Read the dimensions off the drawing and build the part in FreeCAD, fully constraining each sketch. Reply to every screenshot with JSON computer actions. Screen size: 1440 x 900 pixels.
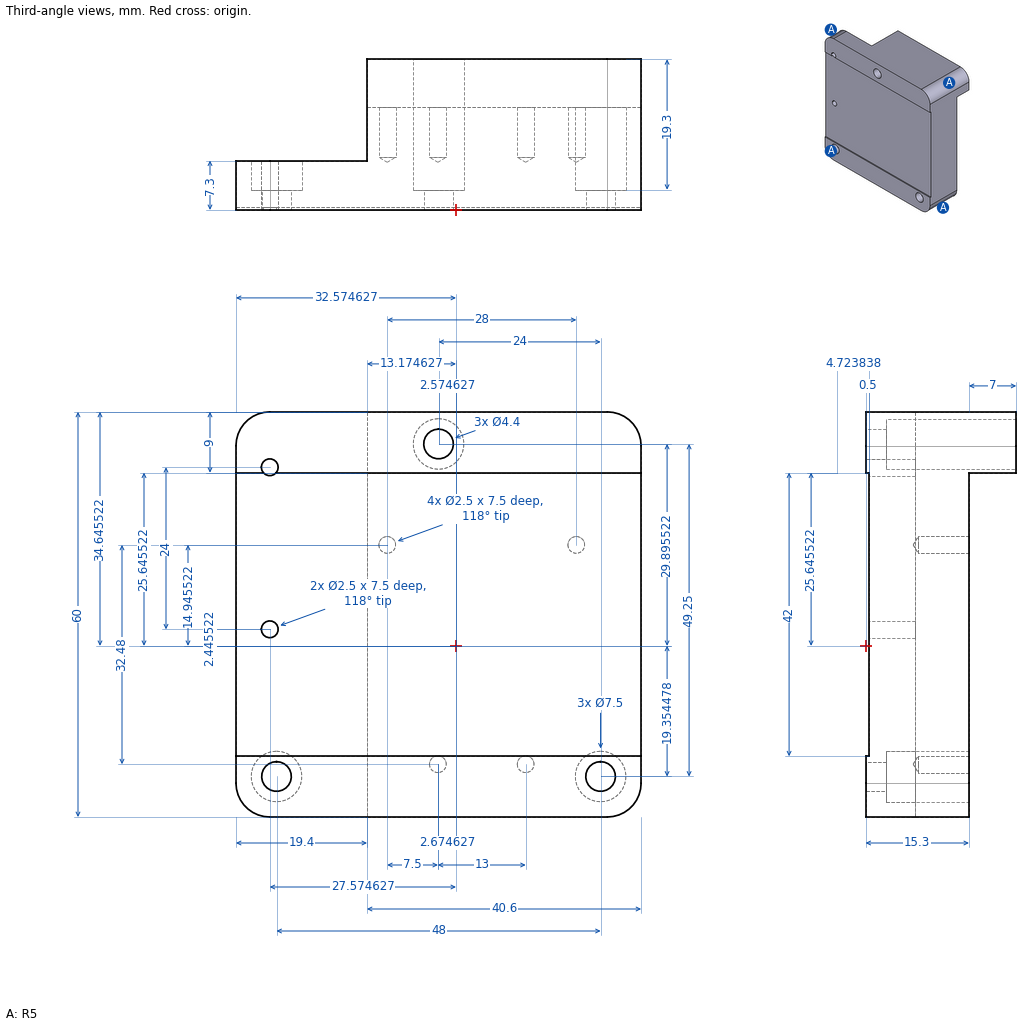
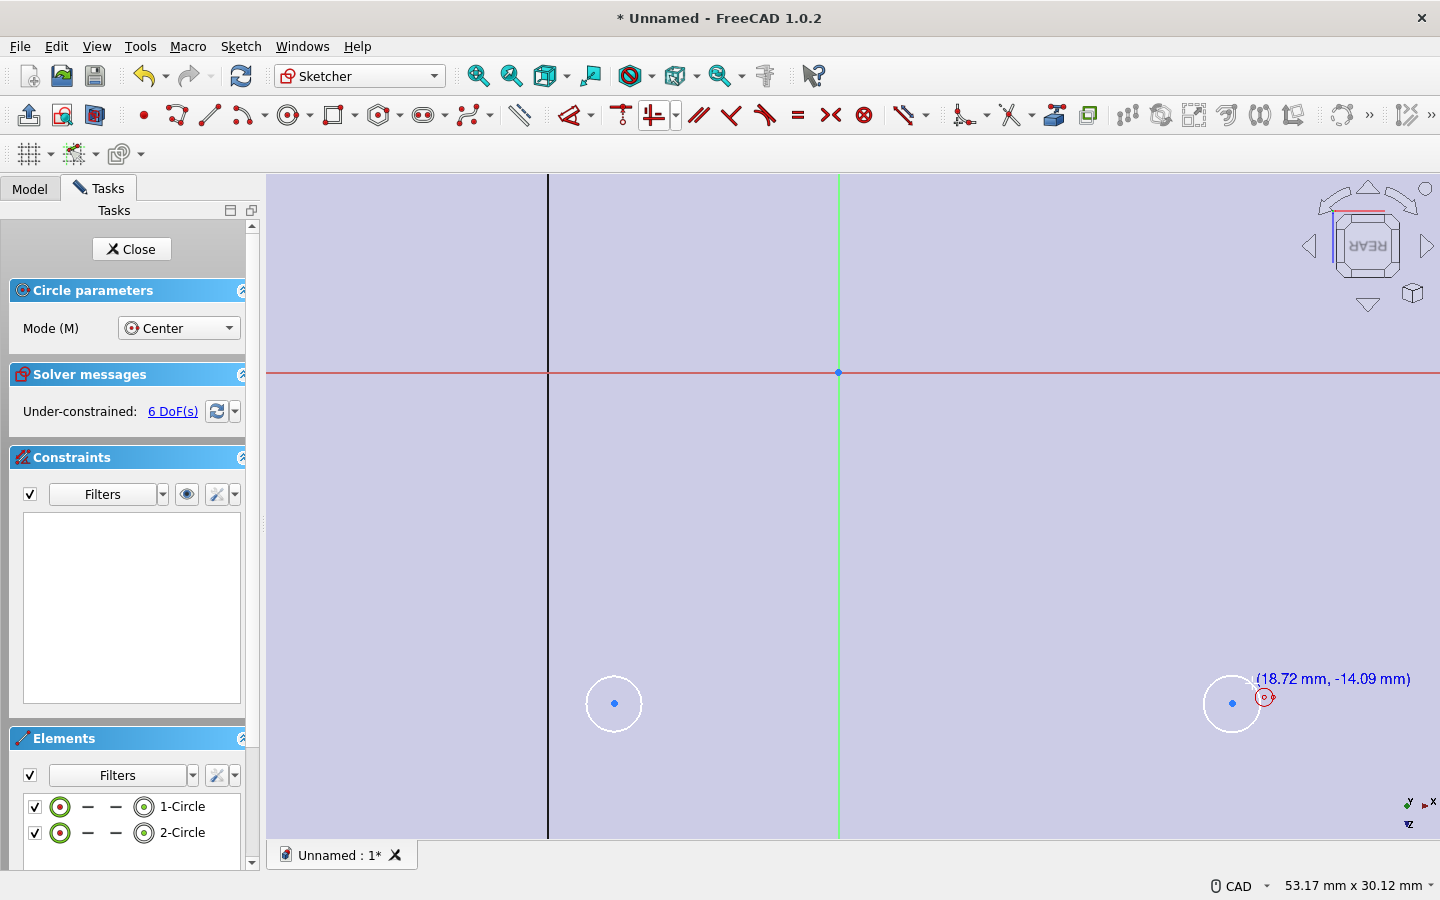
{"action": "scroll", "coordinate": [616, 704], "scroll_direction": "down", "scroll_amount": 3}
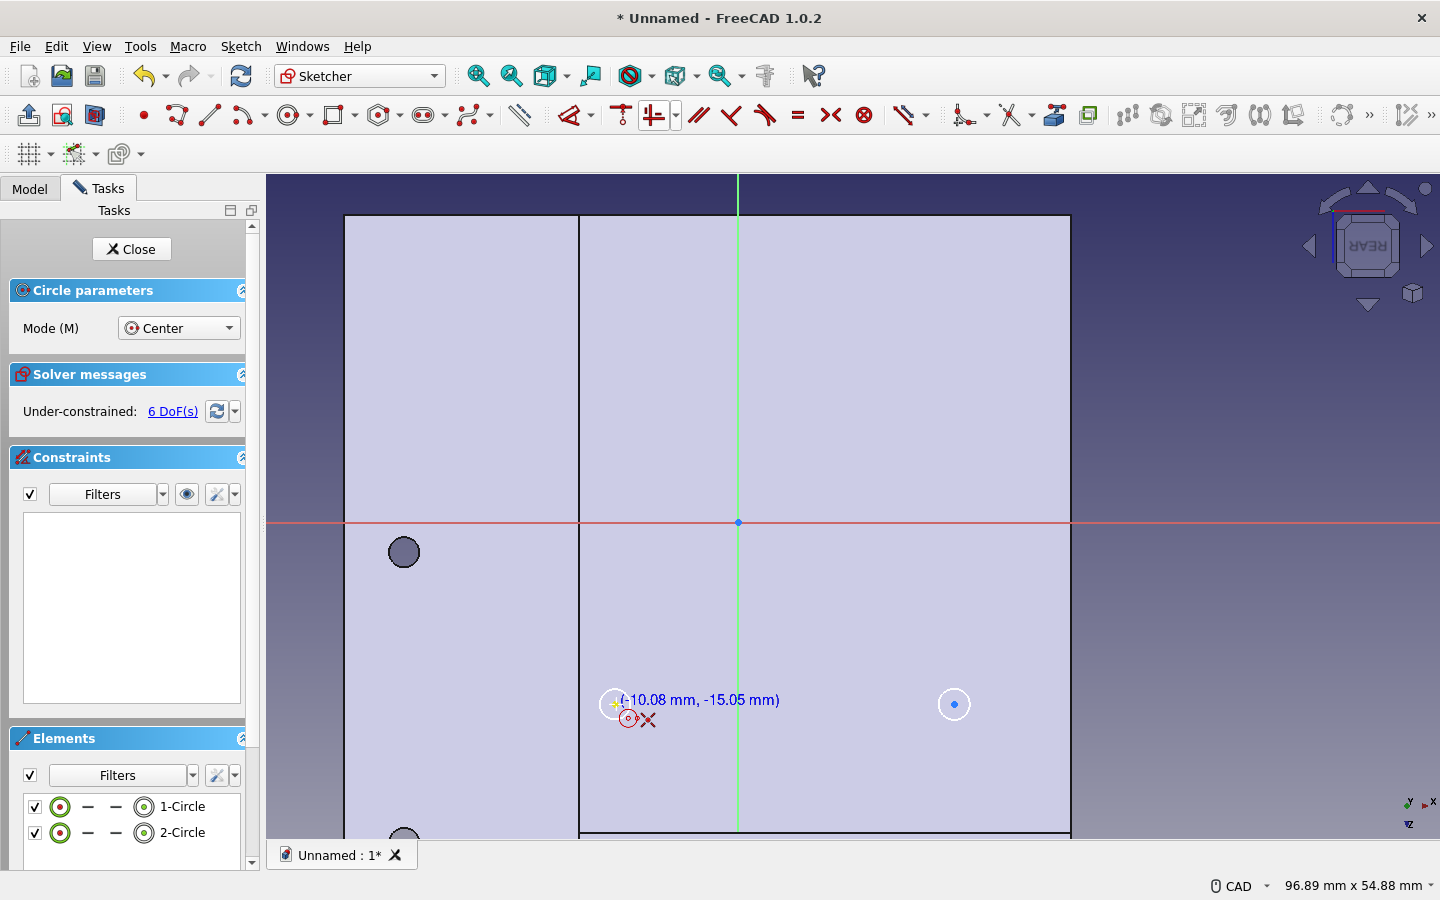
{"action": "scroll", "coordinate": [706, 310], "scroll_direction": "up", "scroll_amount": 3}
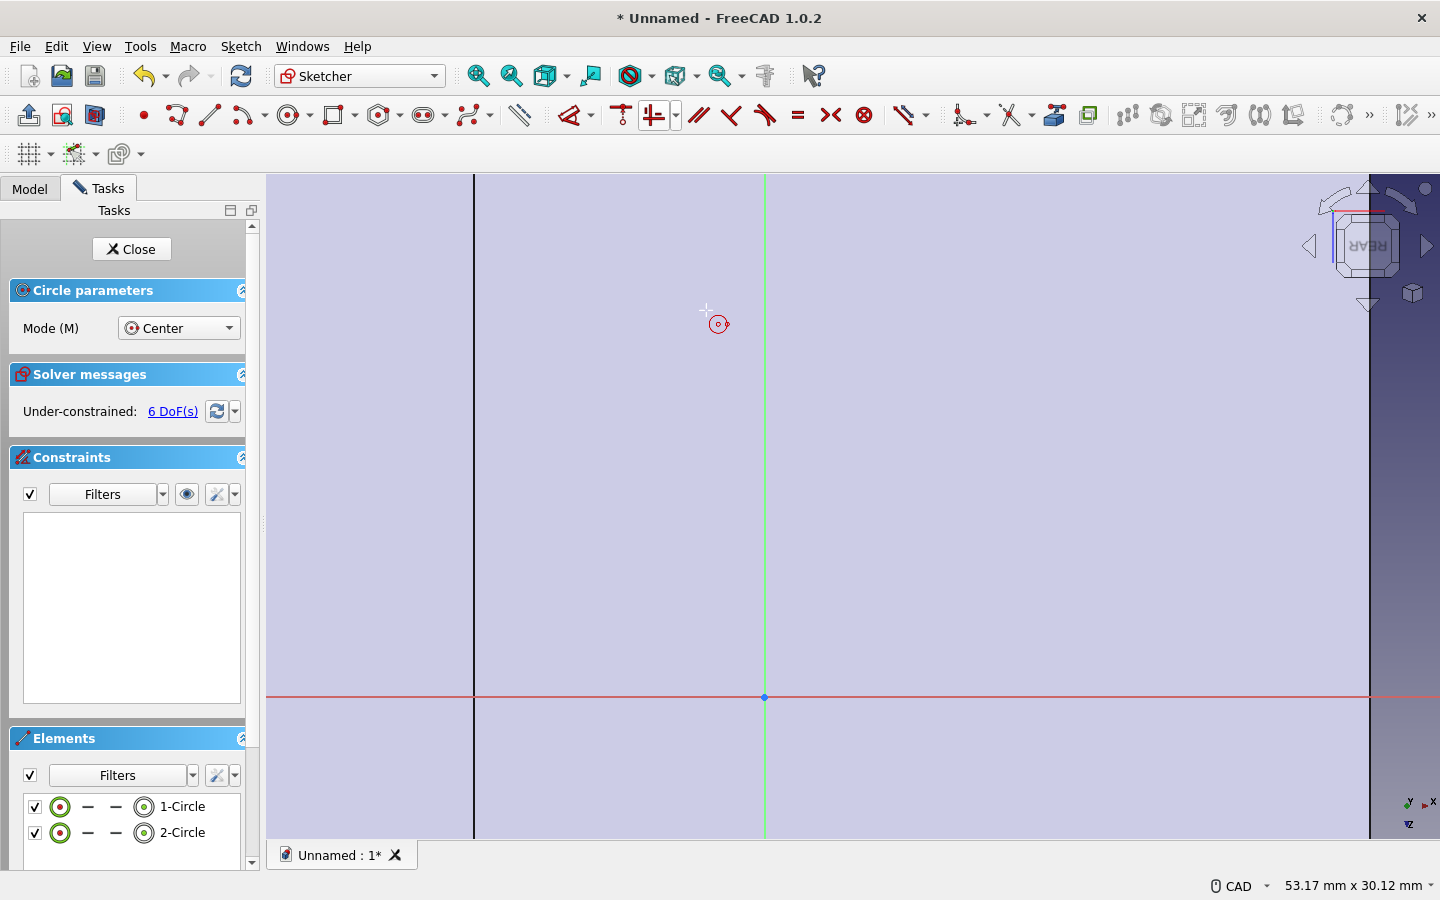
{"action": "left_click", "coordinate": [705, 310]}
{"action": "left_click", "coordinate": [725, 291]}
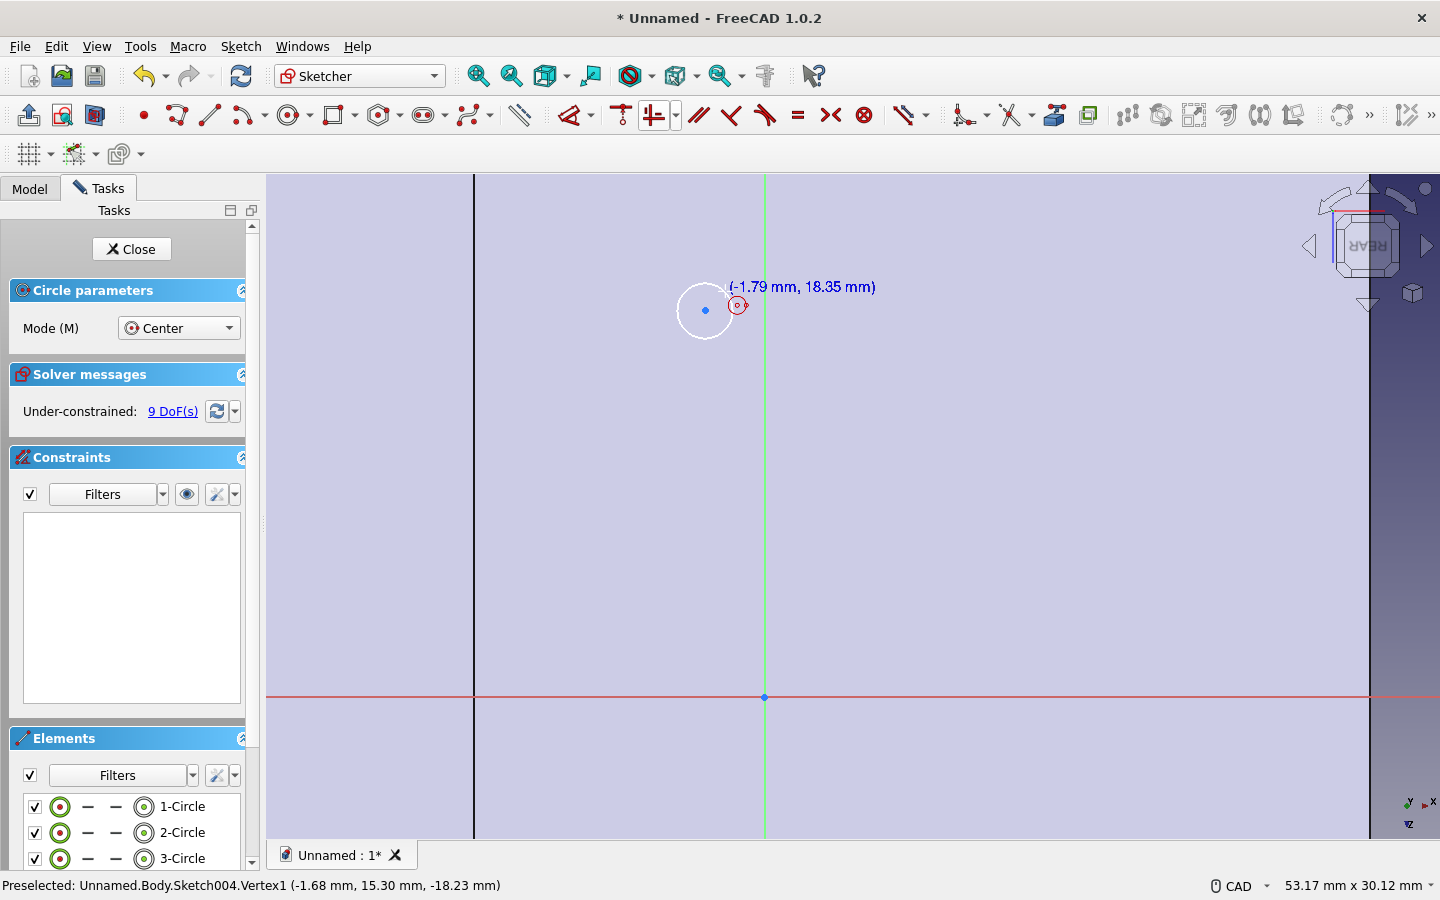
{"action": "left_click", "coordinate": [993, 310]}
{"action": "left_click", "coordinate": [1012, 291]}
{"action": "key", "text": "Escape"}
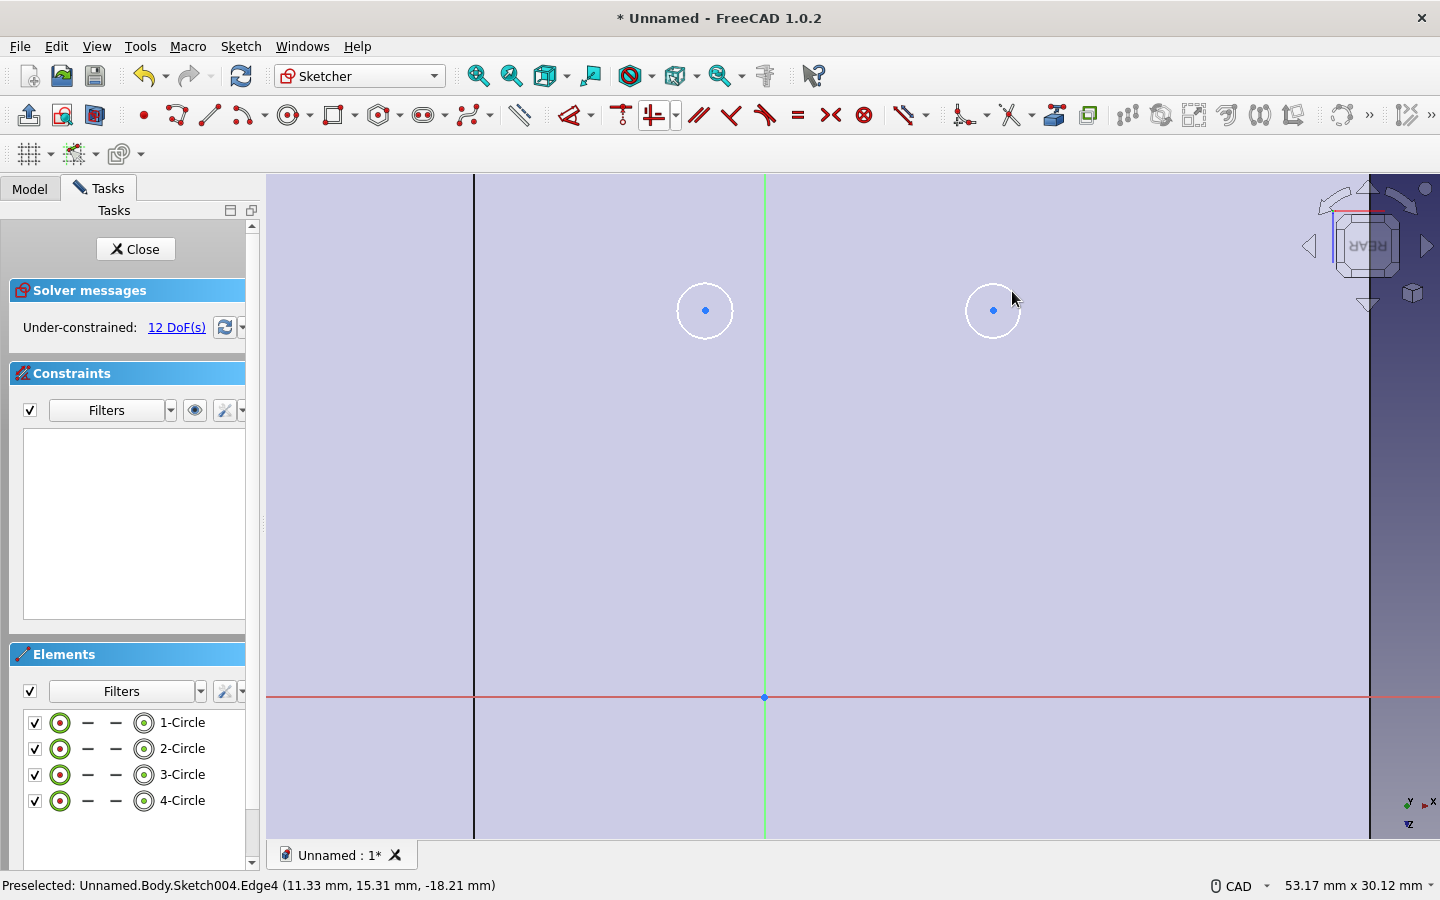
{"action": "scroll", "coordinate": [706, 309], "scroll_direction": "down", "scroll_amount": 3}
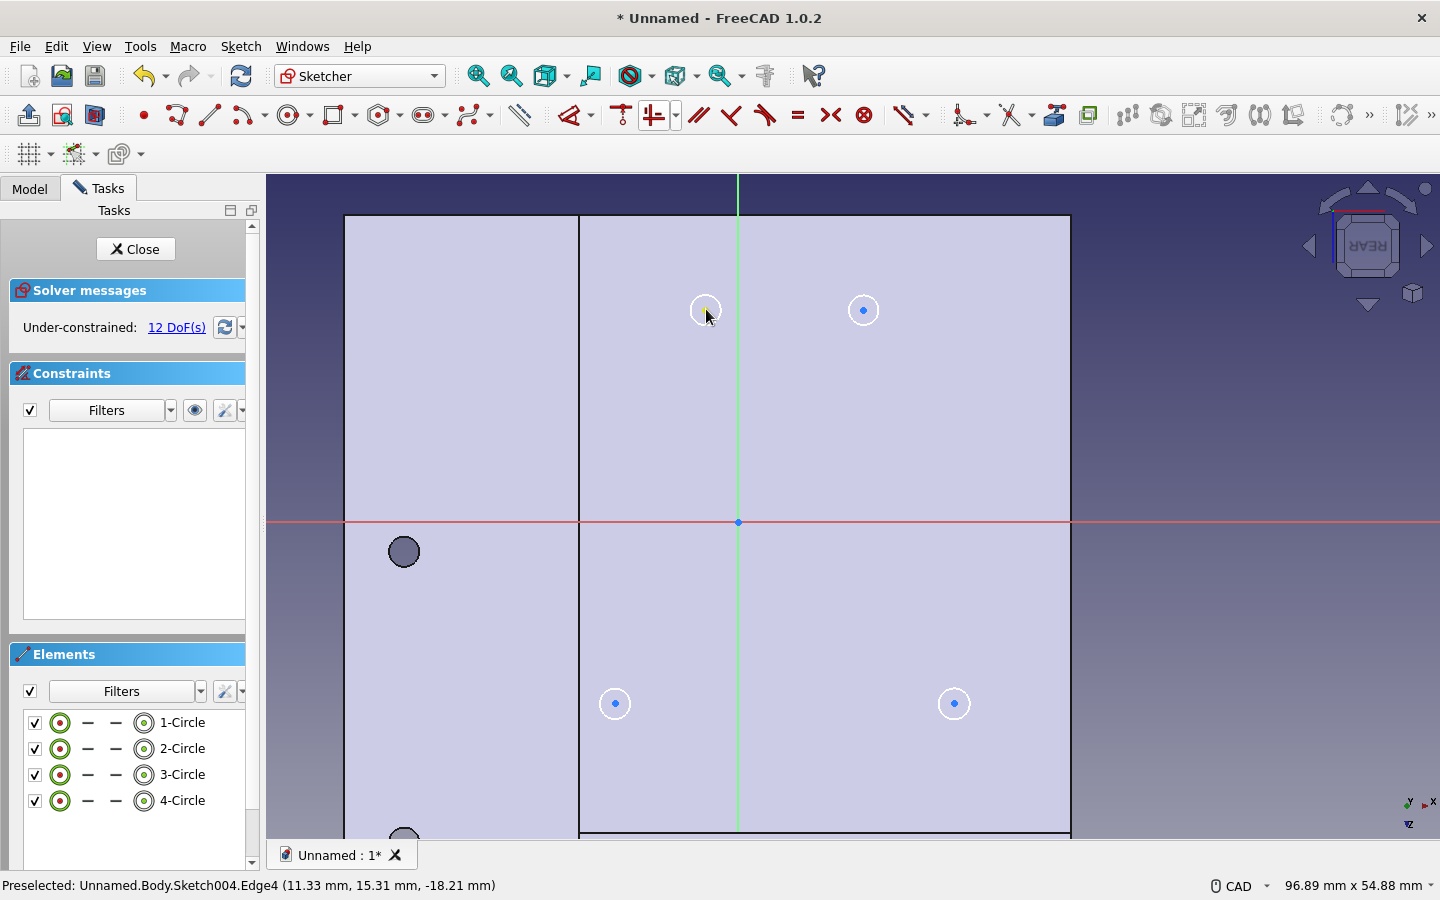
{"action": "left_click", "coordinate": [626, 693]}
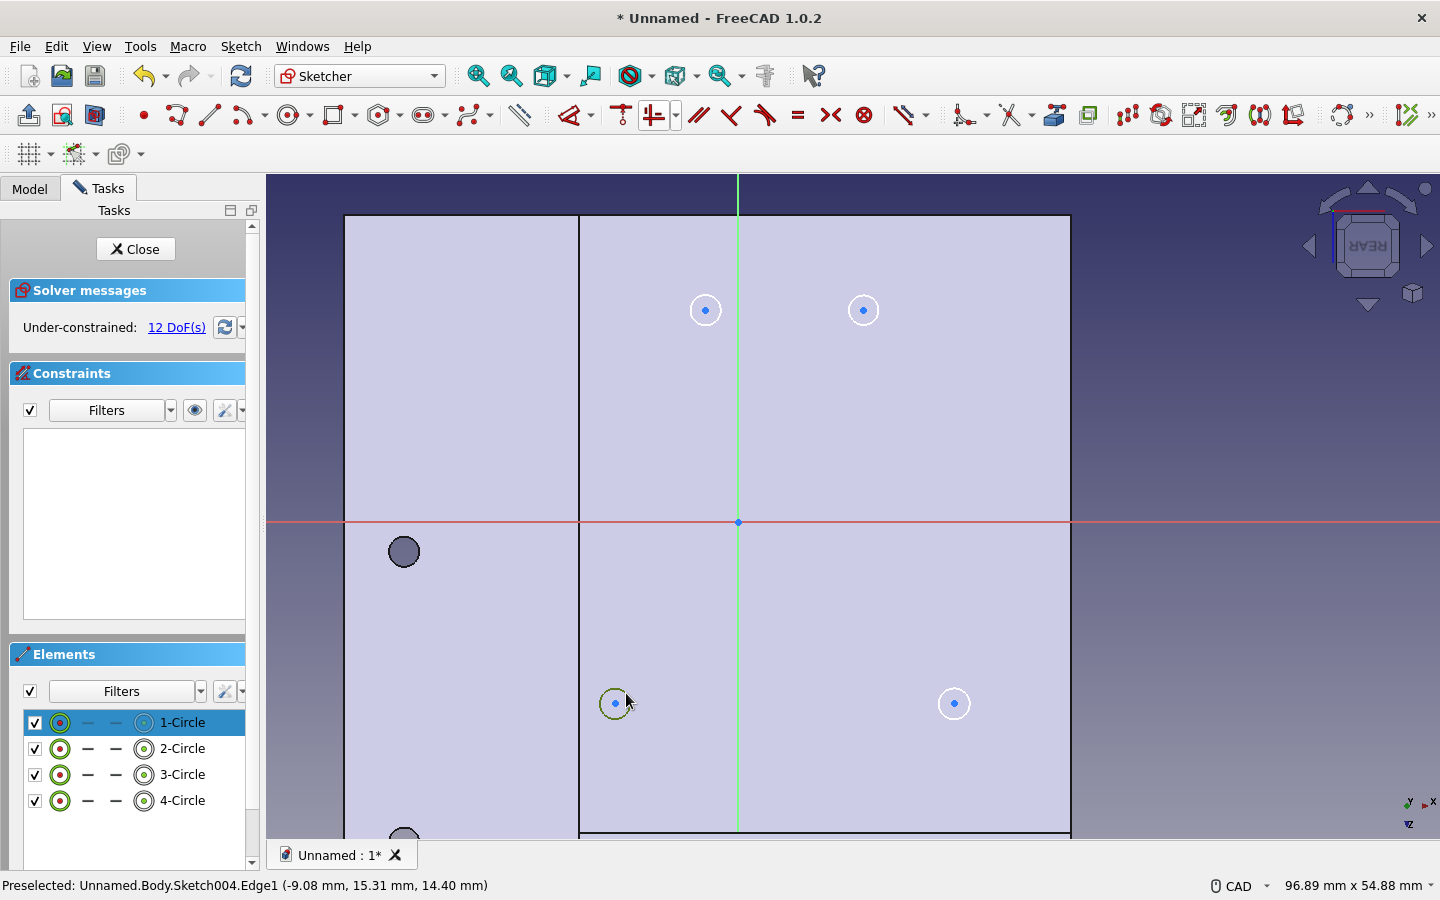
{"action": "left_click", "coordinate": [965, 693]}